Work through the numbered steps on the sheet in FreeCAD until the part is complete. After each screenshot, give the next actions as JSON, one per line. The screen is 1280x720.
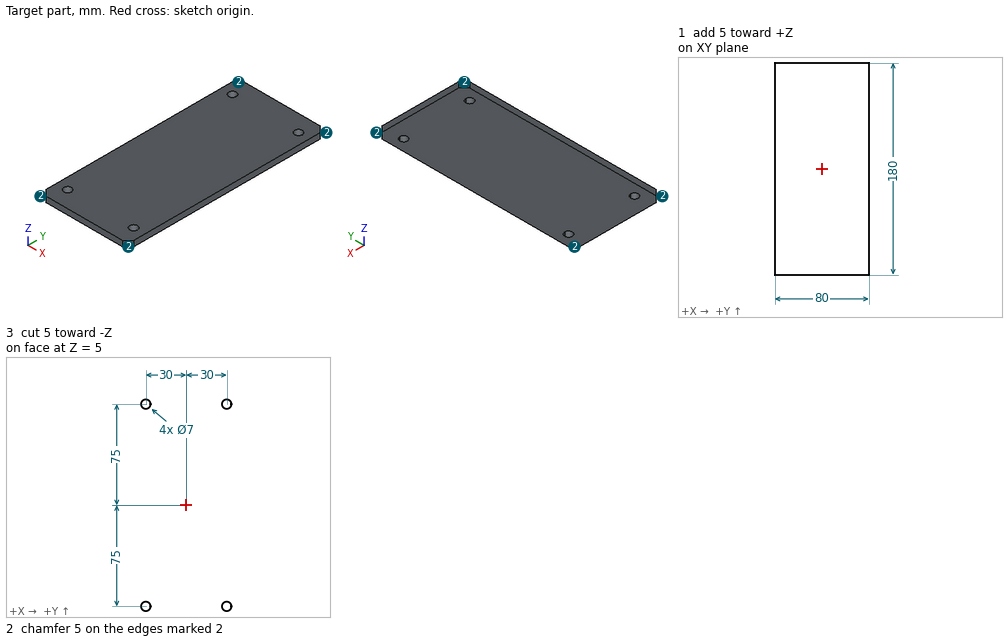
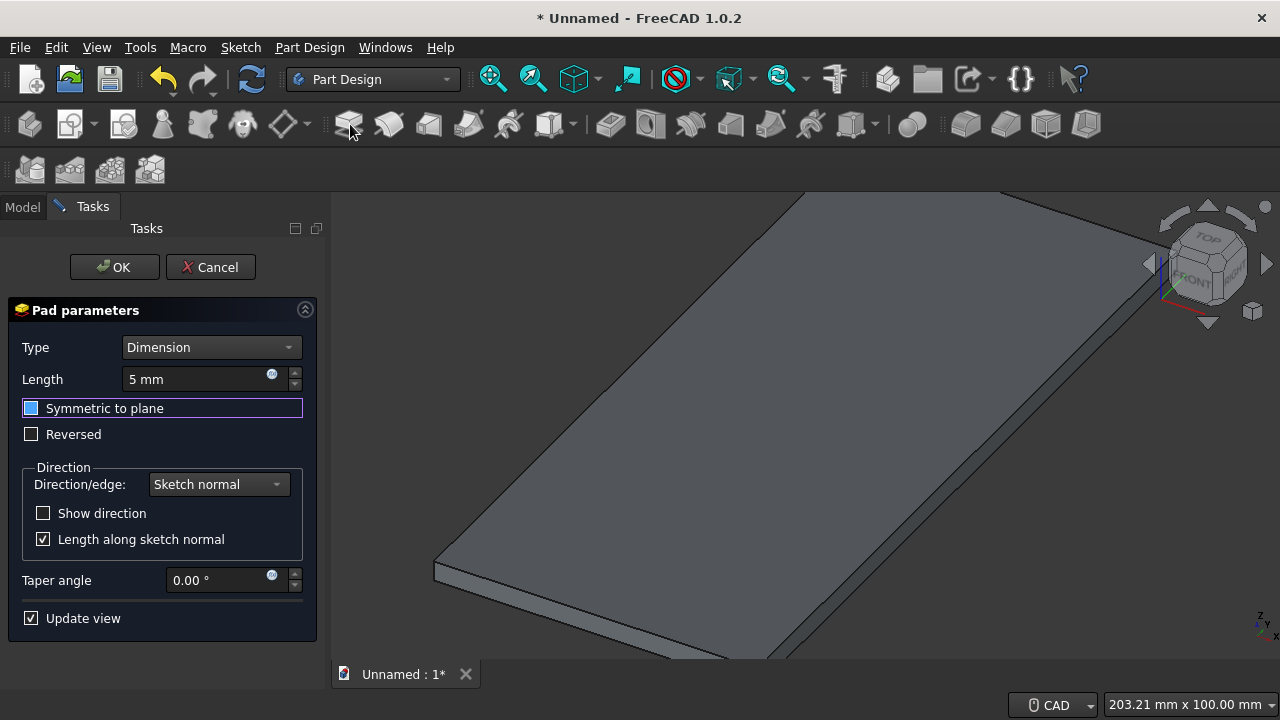
{"action": "left_click", "coordinate": [115, 267]}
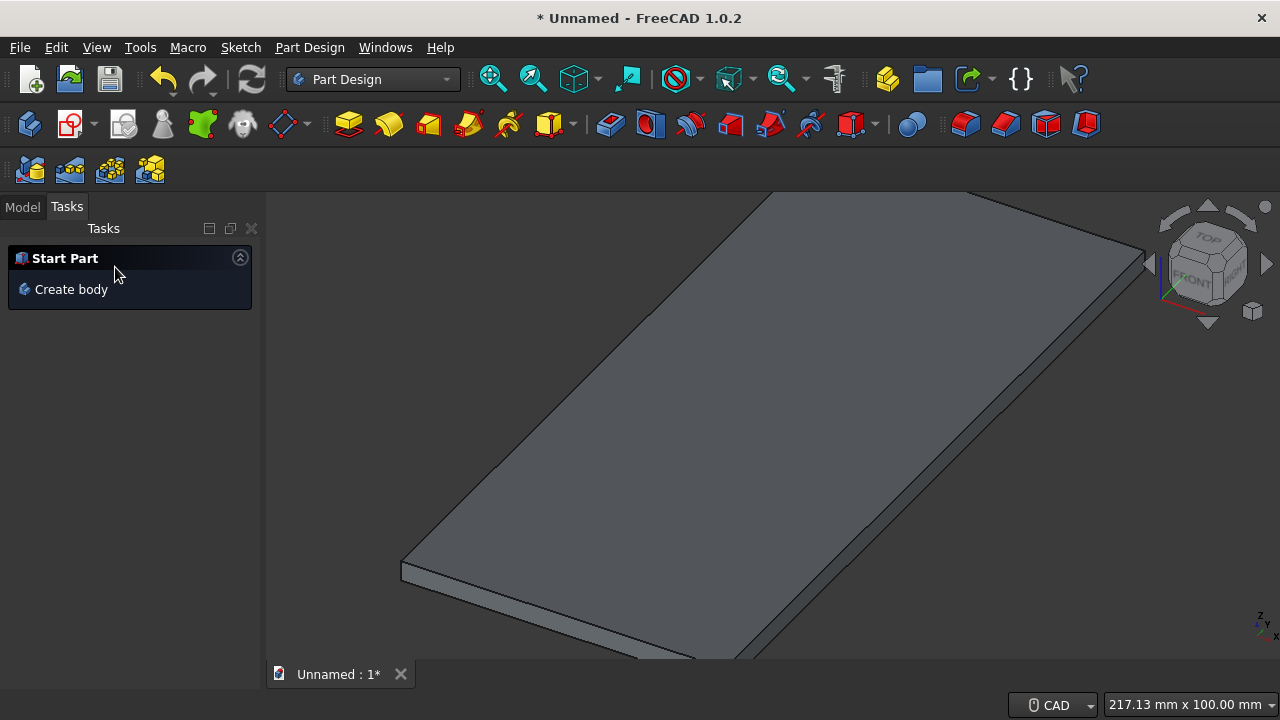
{"action": "left_click", "coordinate": [494, 80]}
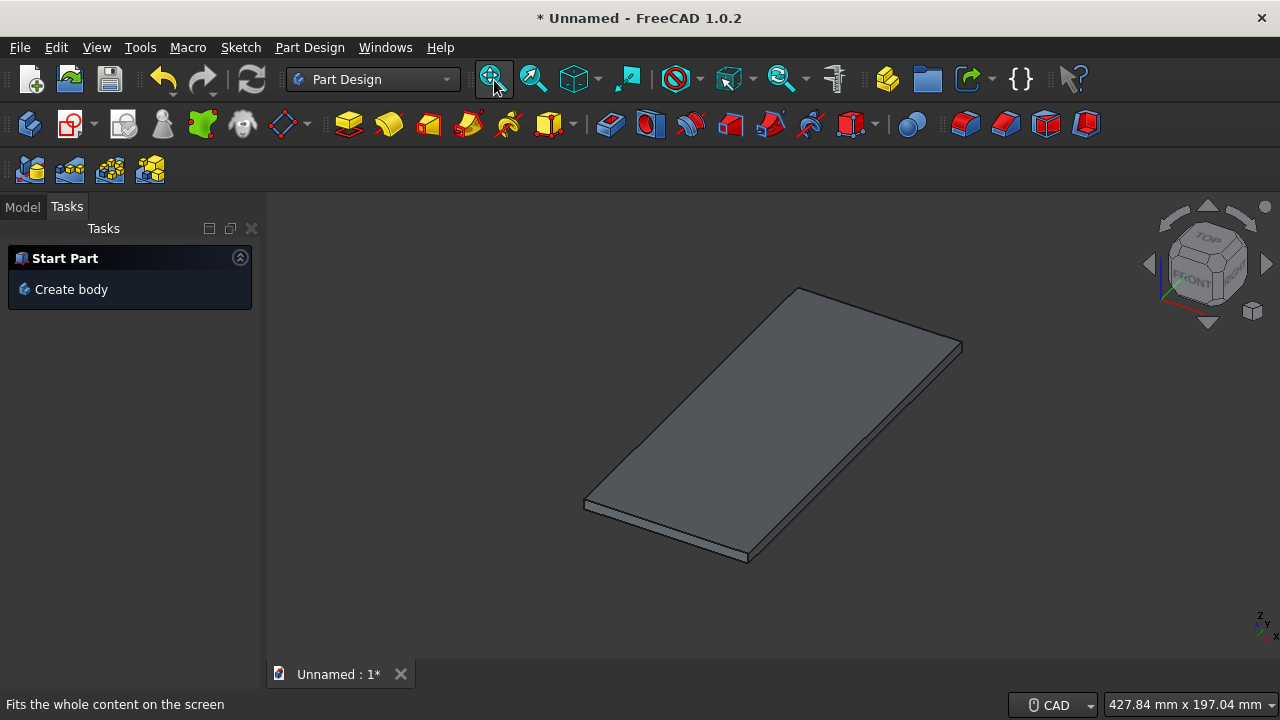
{"action": "left_click", "coordinate": [748, 559]}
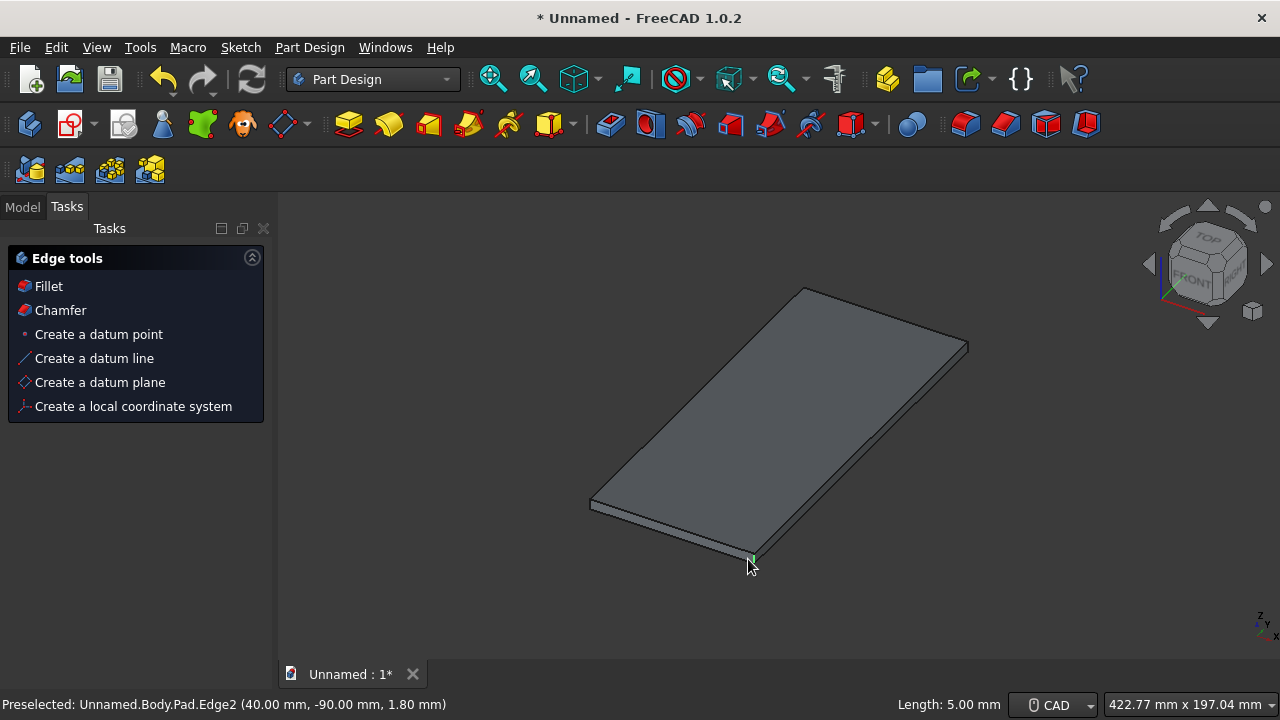
{"action": "scroll", "coordinate": [590, 503], "scroll_direction": "up", "scroll_amount": 7}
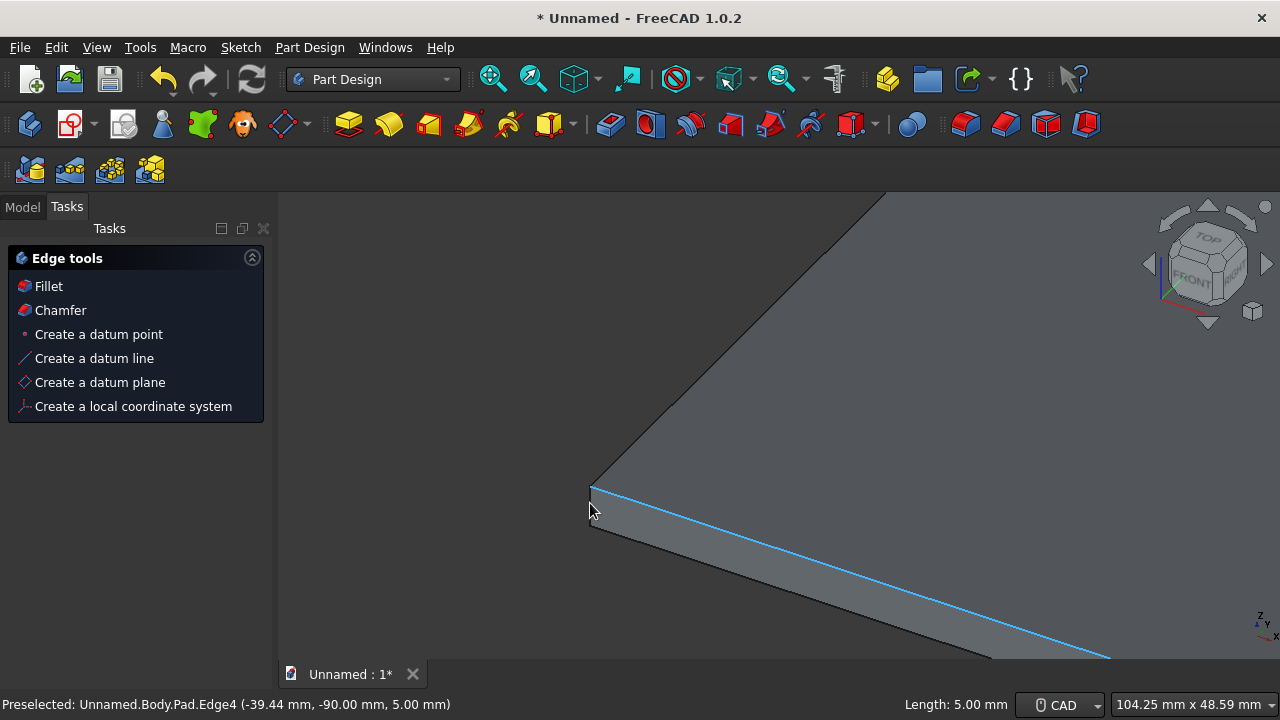
{"action": "left_click", "coordinate": [494, 80]}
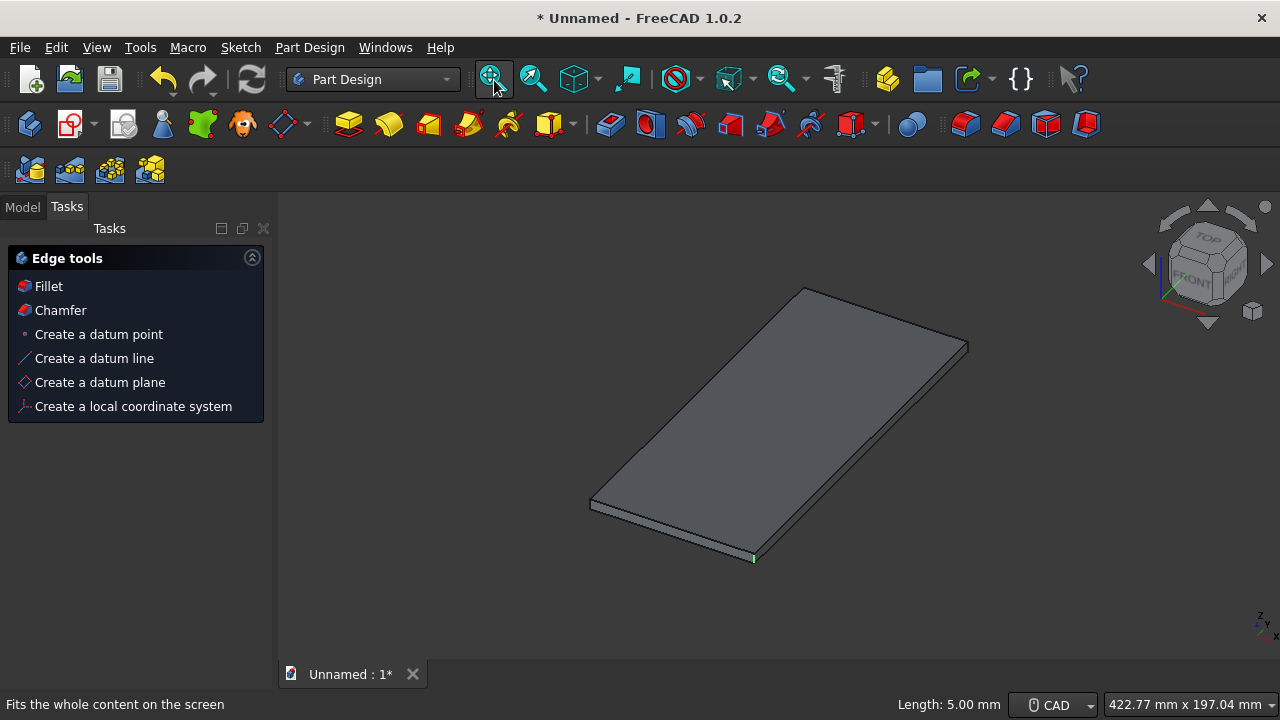
{"action": "key", "text": "0"}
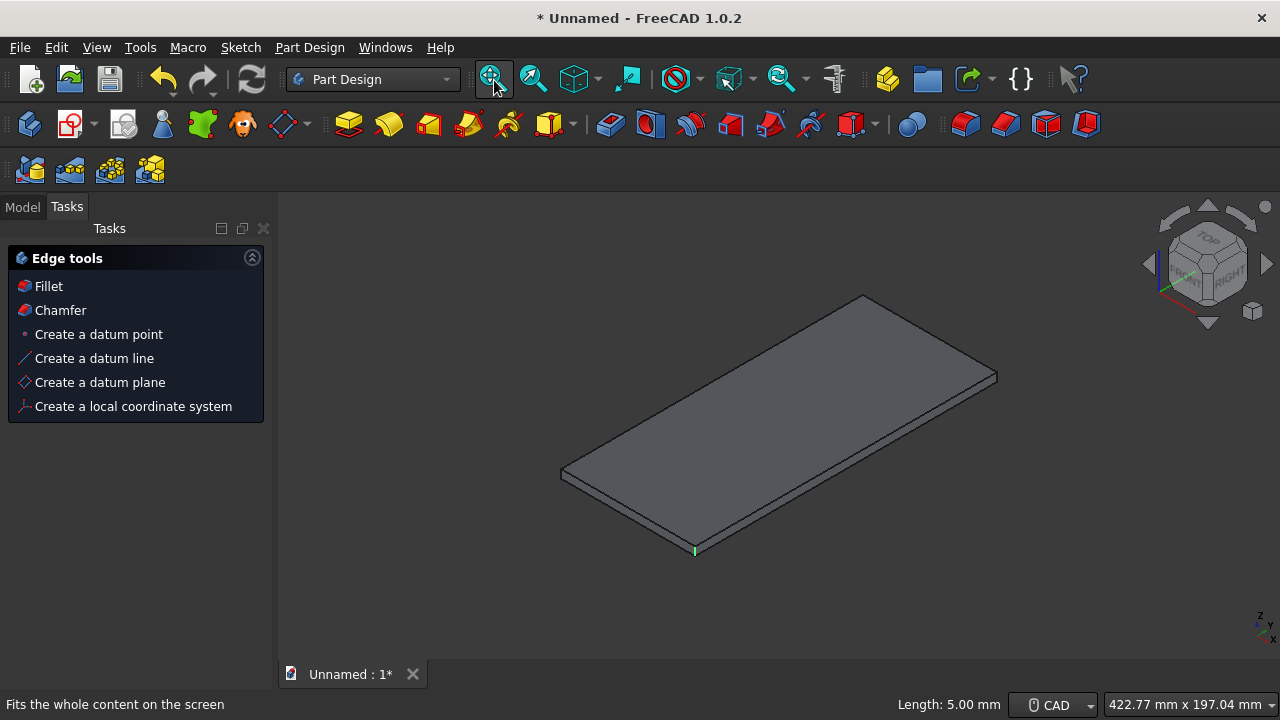
{"action": "scroll", "coordinate": [561, 473], "scroll_direction": "up", "scroll_amount": 7}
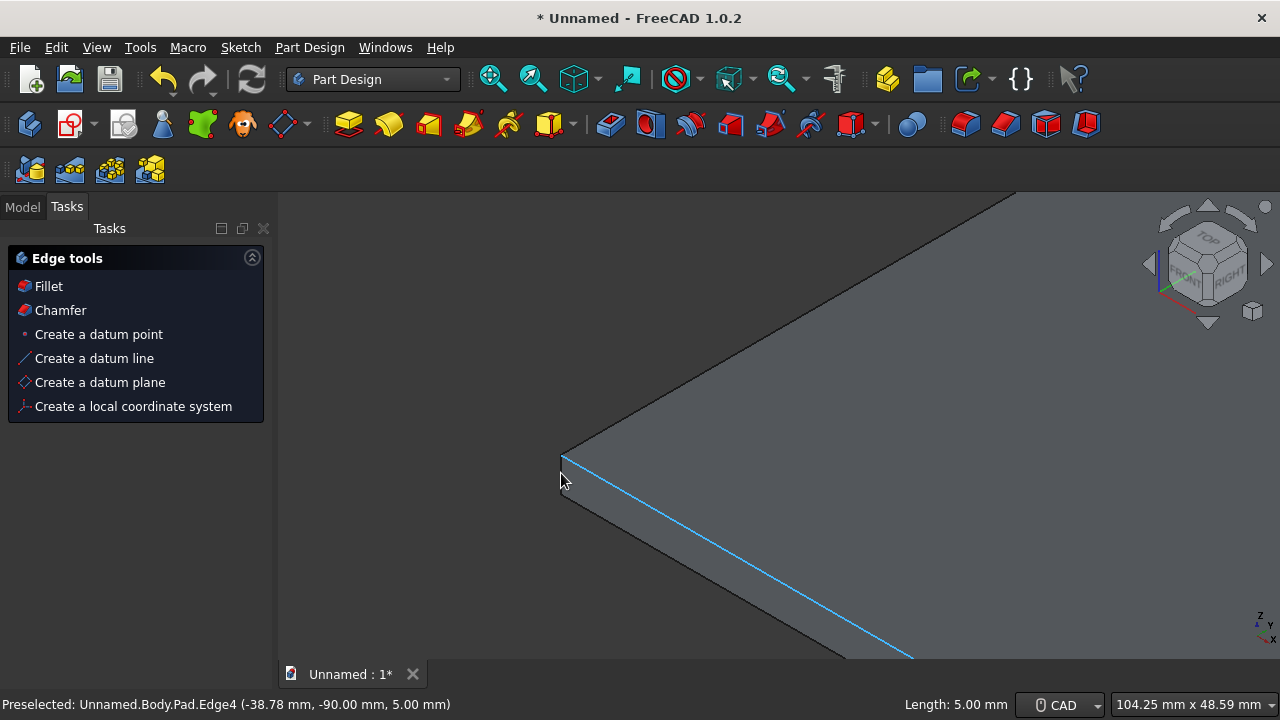
{"action": "left_click", "coordinate": [494, 80]}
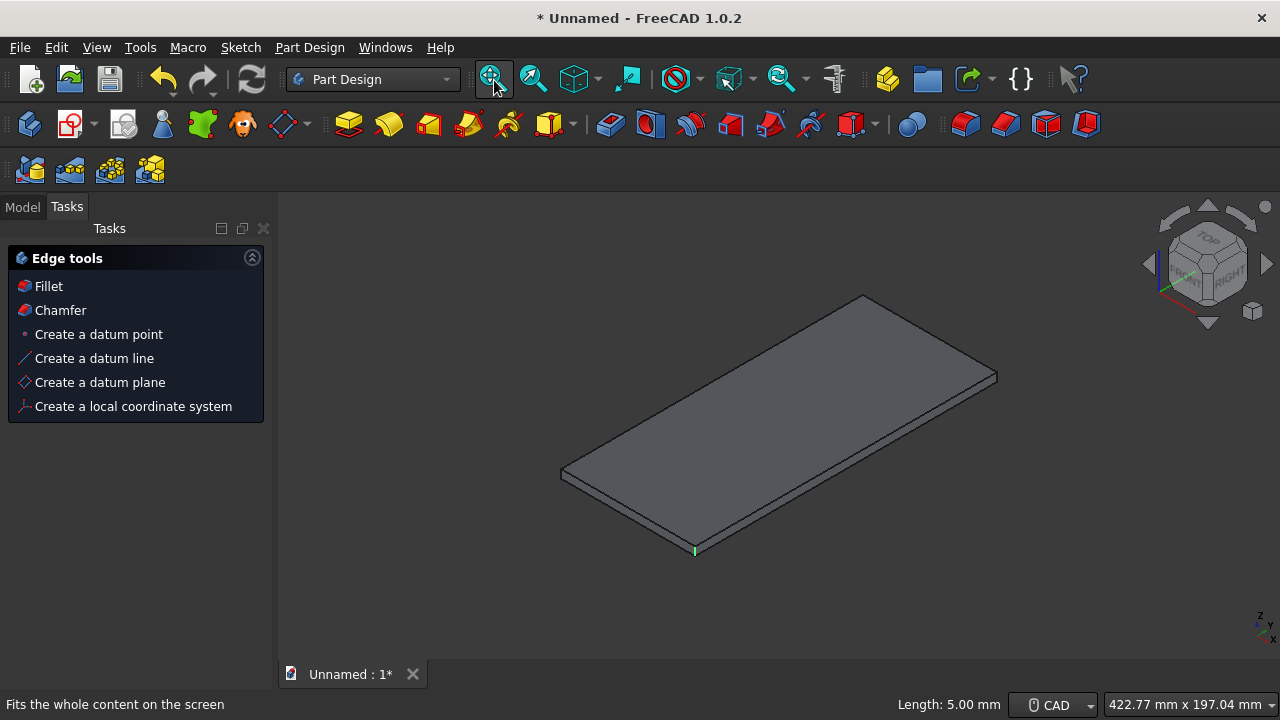
{"action": "key", "text": "2"}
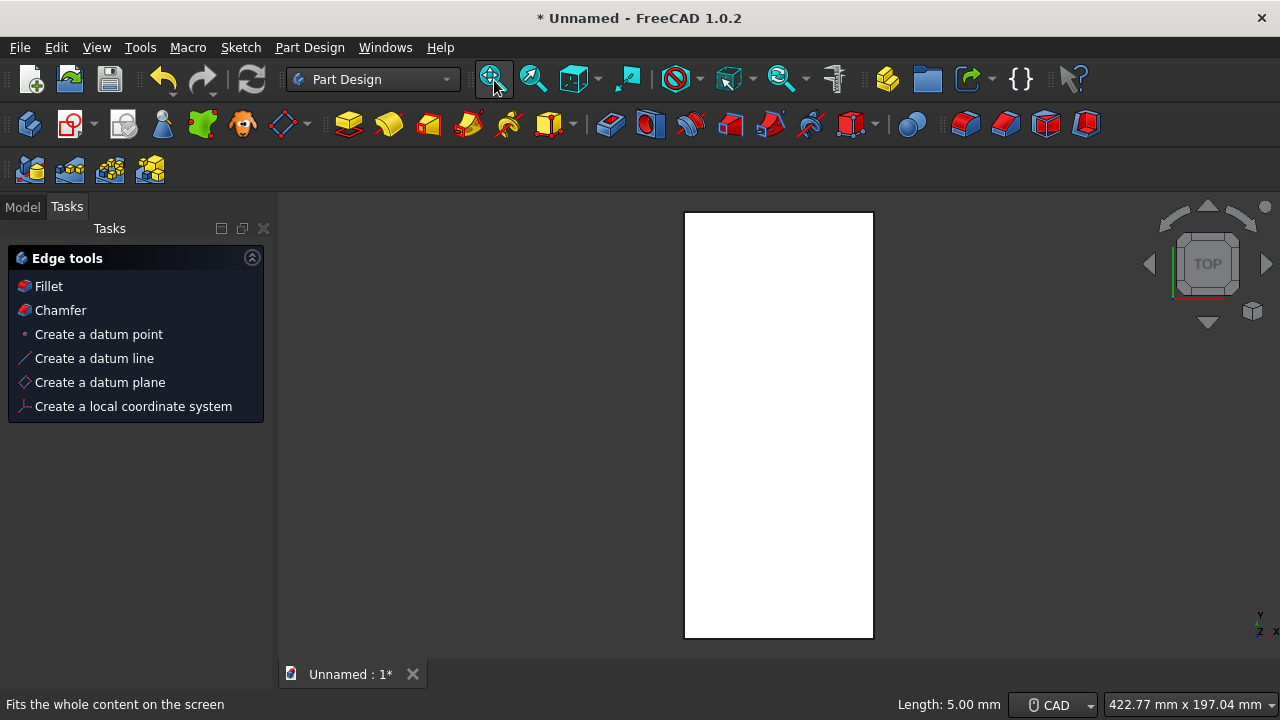
{"action": "key", "text": "1"}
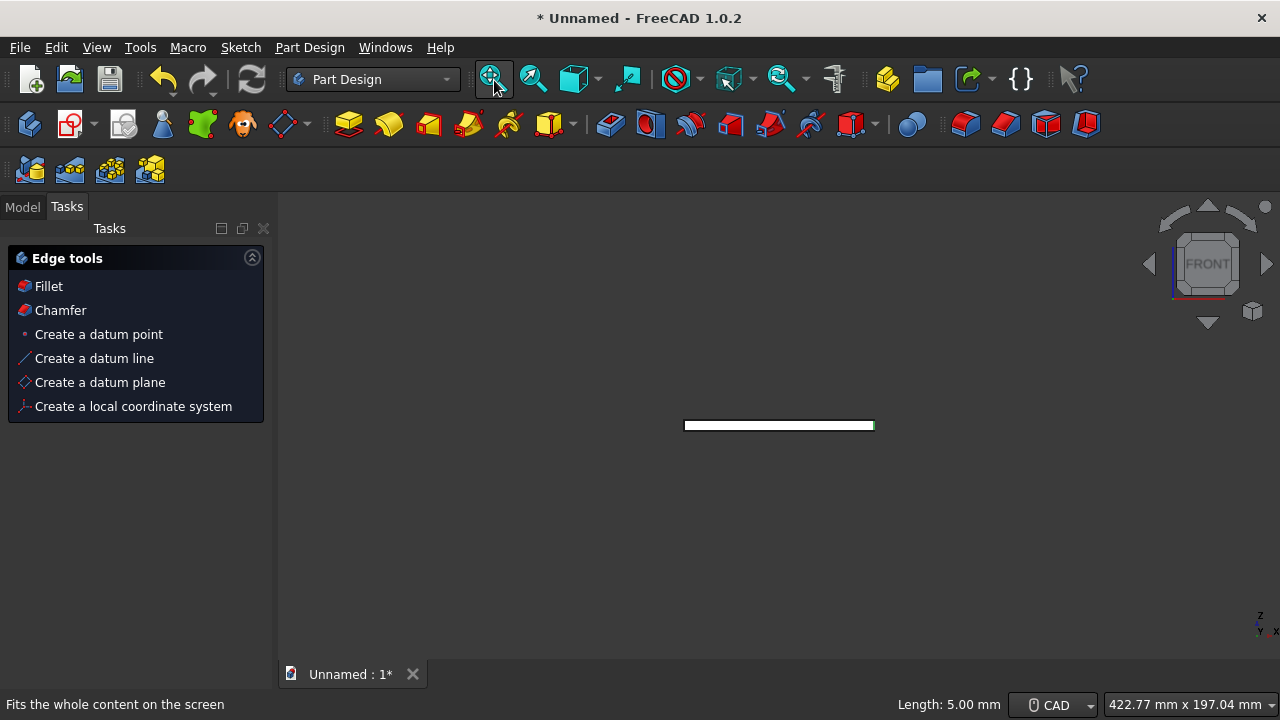
{"action": "left_click", "coordinate": [494, 80]}